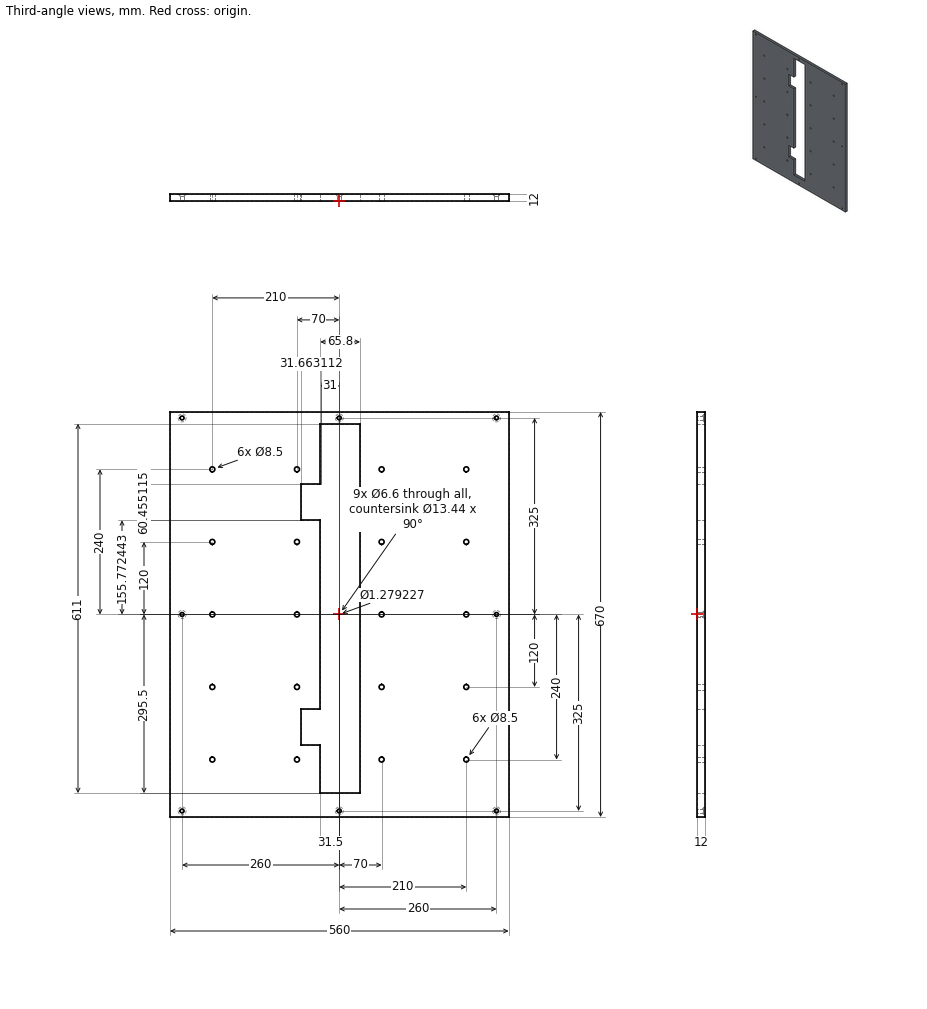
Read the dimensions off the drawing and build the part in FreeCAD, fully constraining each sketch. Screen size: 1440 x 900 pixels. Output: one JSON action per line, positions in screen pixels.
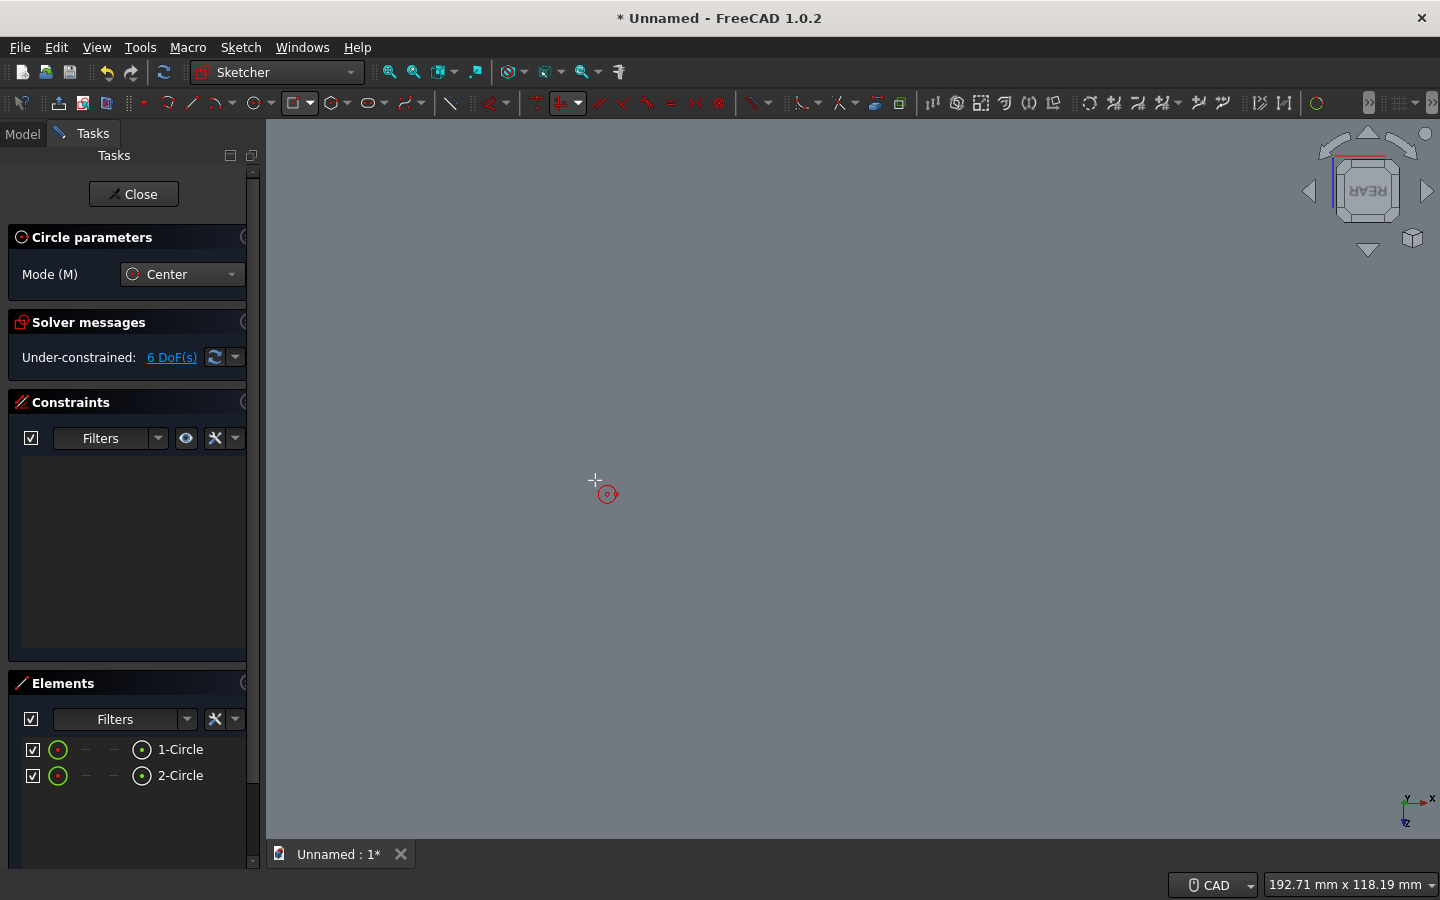
{"action": "left_click", "coordinate": [595, 478]}
{"action": "left_click", "coordinate": [614, 460]}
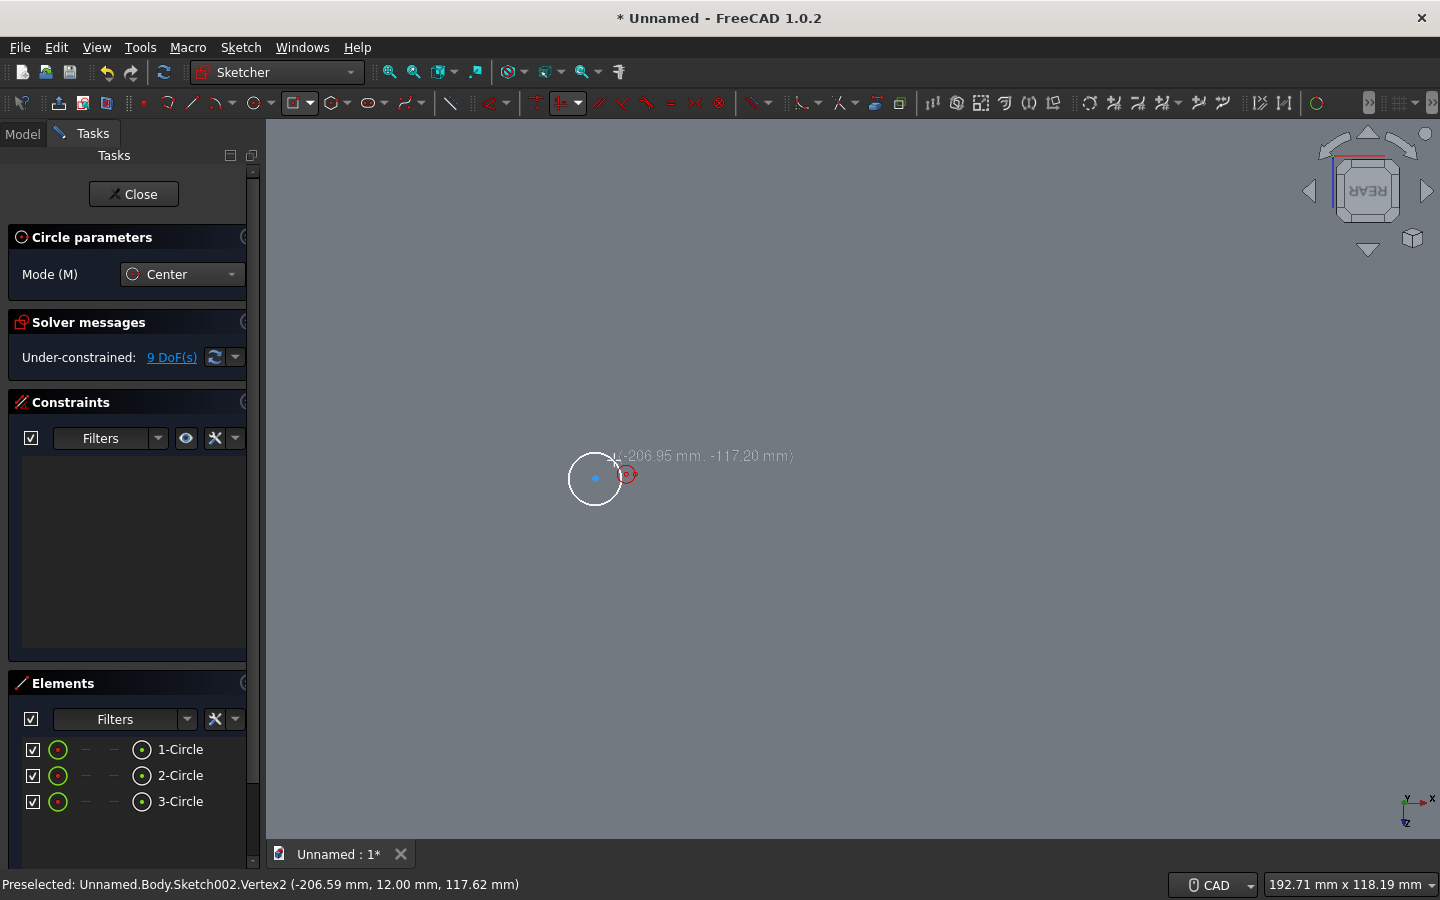
{"action": "scroll", "coordinate": [595, 479], "scroll_direction": "down", "scroll_amount": 6}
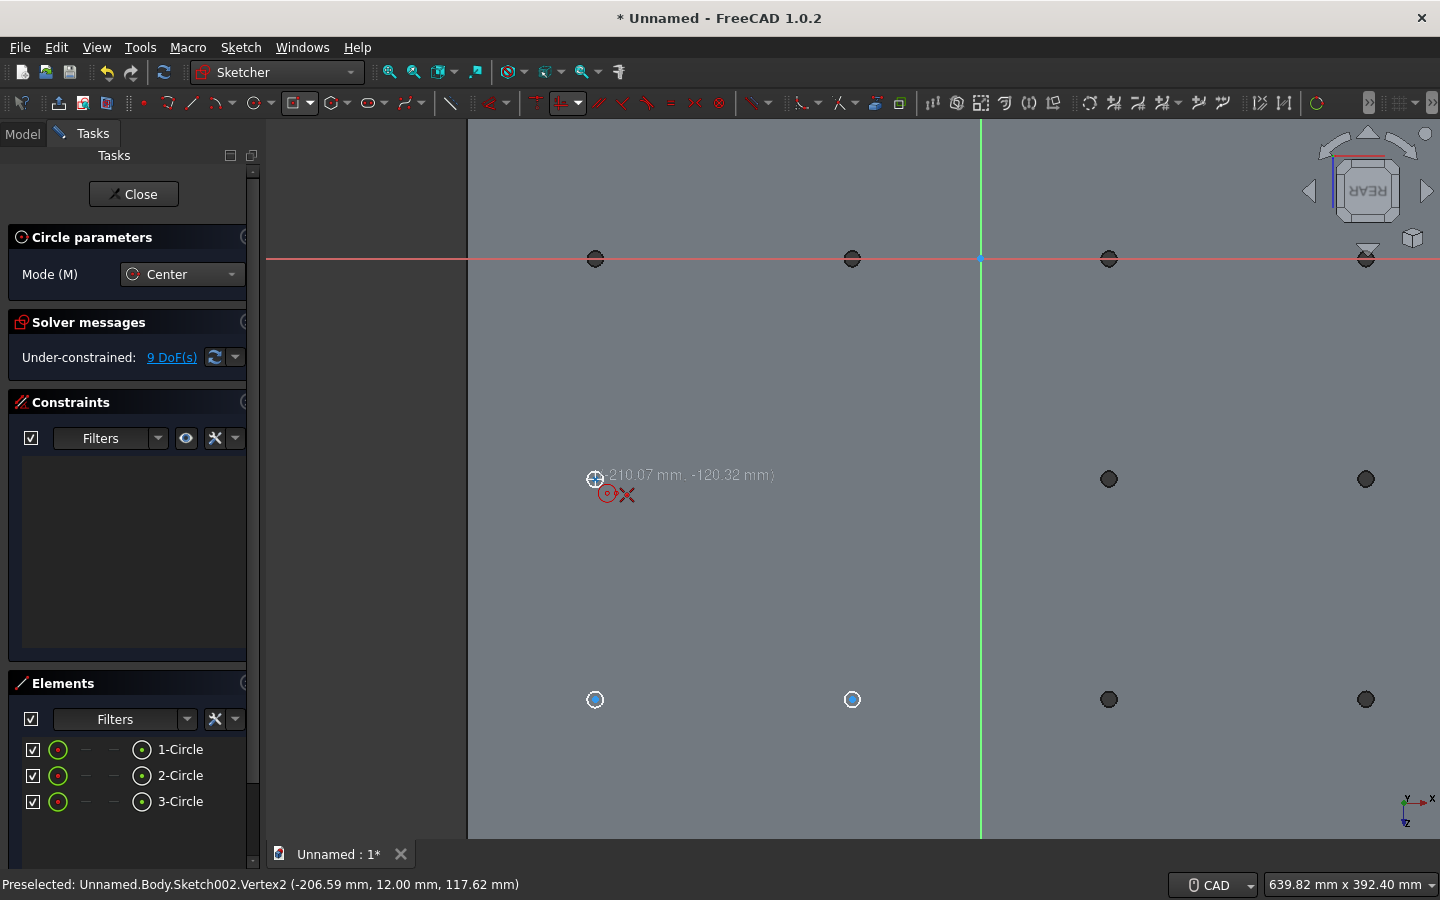
{"action": "scroll", "coordinate": [852, 479], "scroll_direction": "up", "scroll_amount": 6}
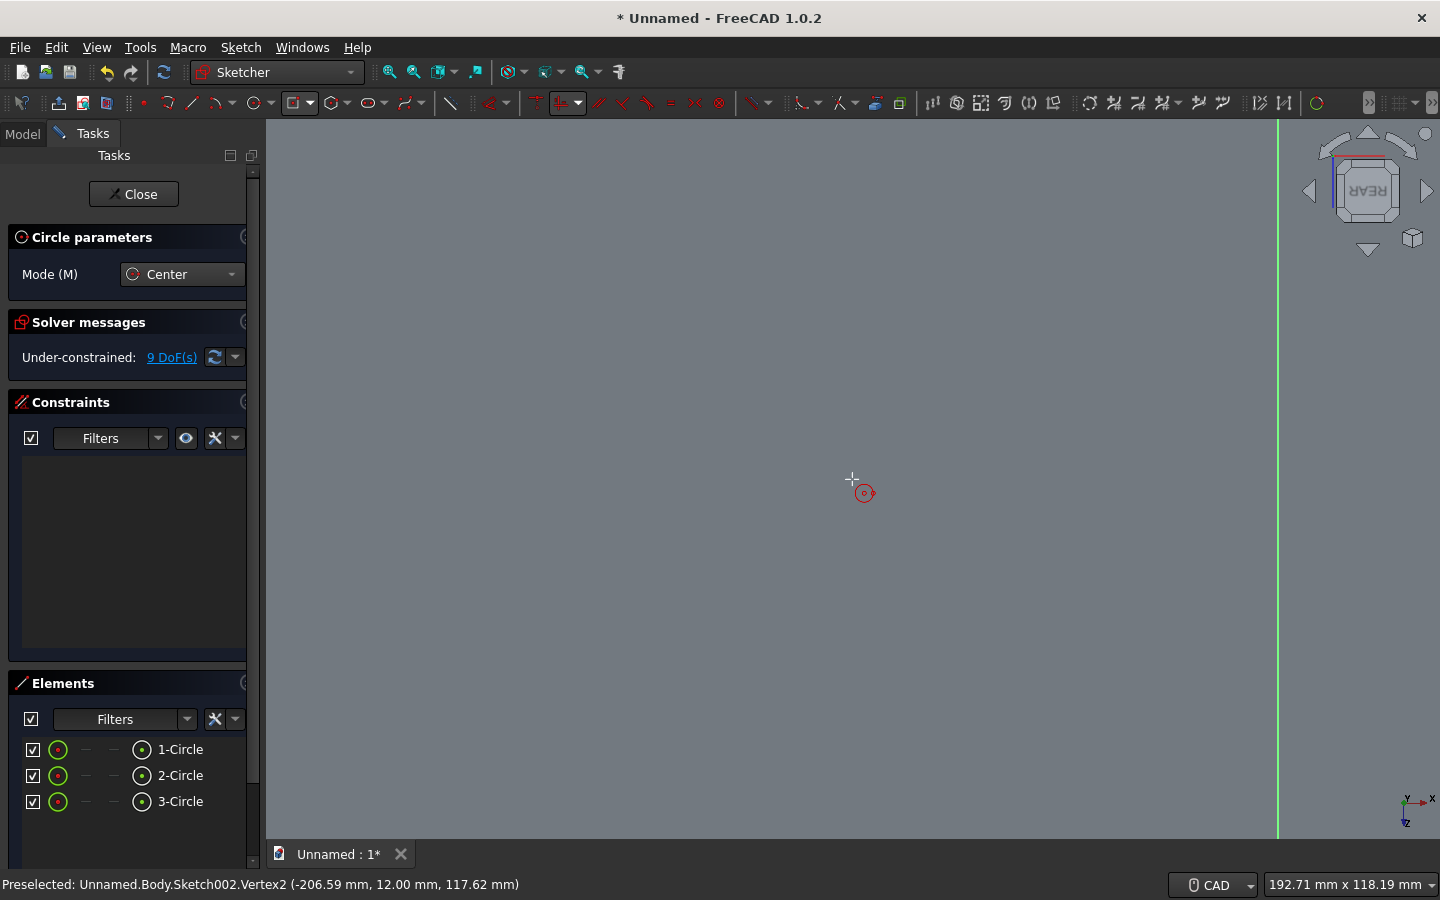
{"action": "left_click", "coordinate": [852, 478]}
{"action": "left_click", "coordinate": [870, 460]}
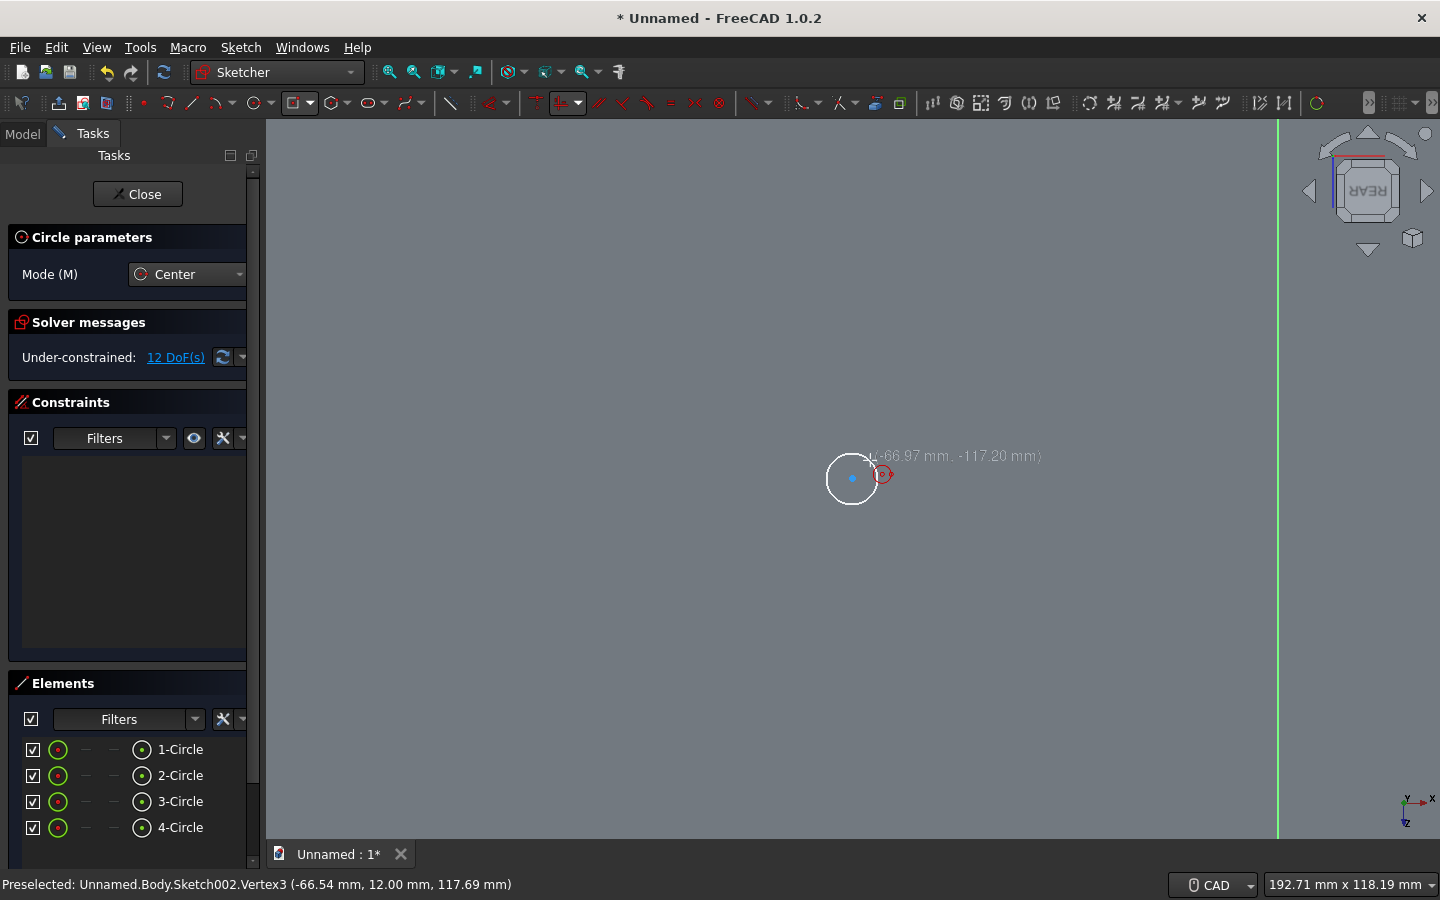
{"action": "scroll", "coordinate": [852, 479], "scroll_direction": "down", "scroll_amount": 6}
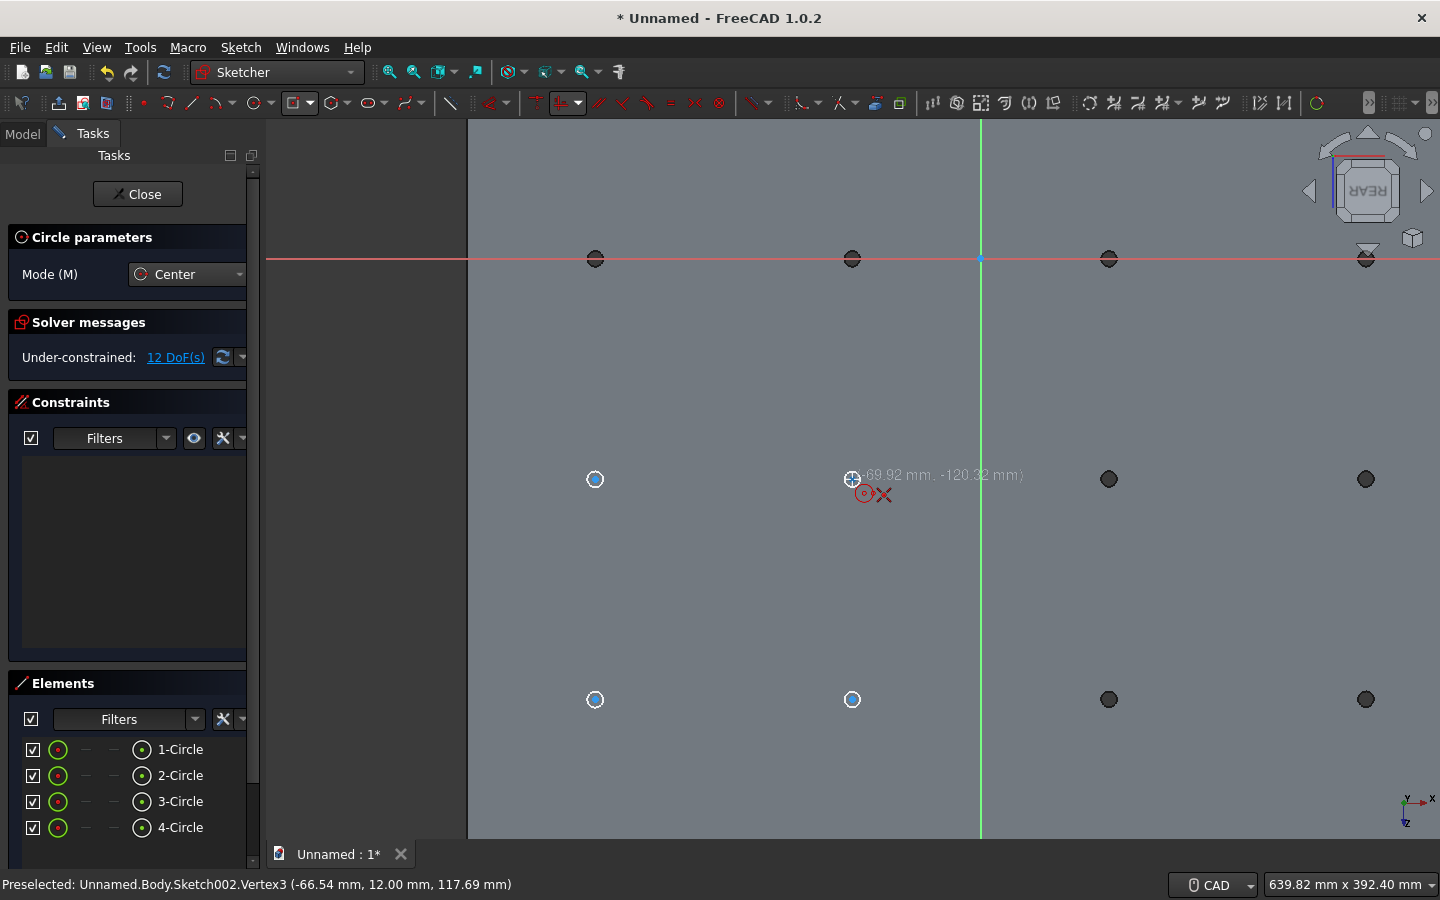
{"action": "scroll", "coordinate": [852, 259], "scroll_direction": "up", "scroll_amount": 6}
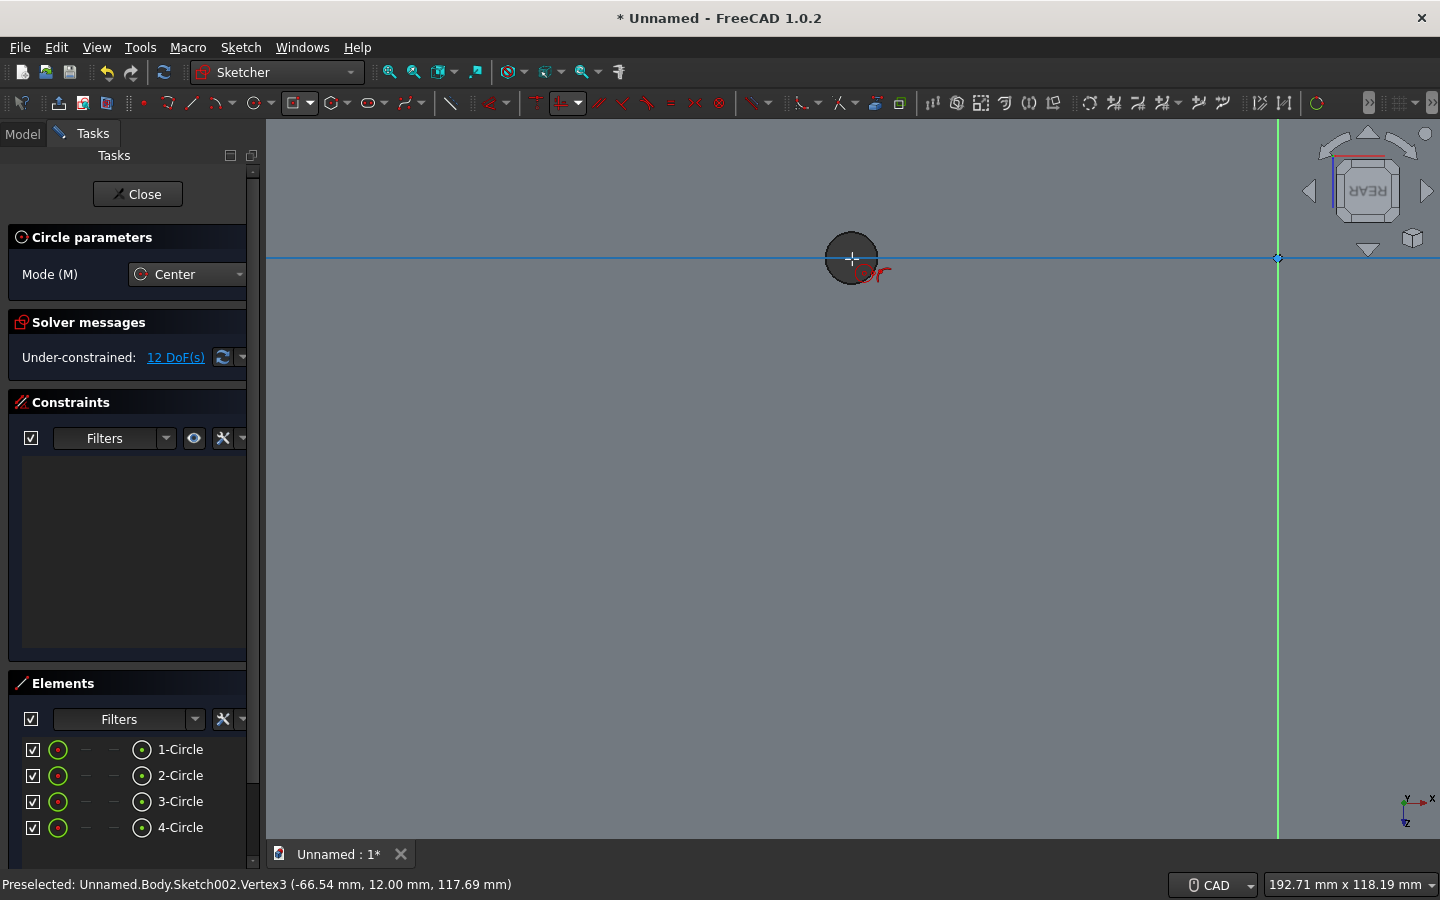
{"action": "left_click", "coordinate": [852, 258]}
{"action": "left_click", "coordinate": [870, 240]}